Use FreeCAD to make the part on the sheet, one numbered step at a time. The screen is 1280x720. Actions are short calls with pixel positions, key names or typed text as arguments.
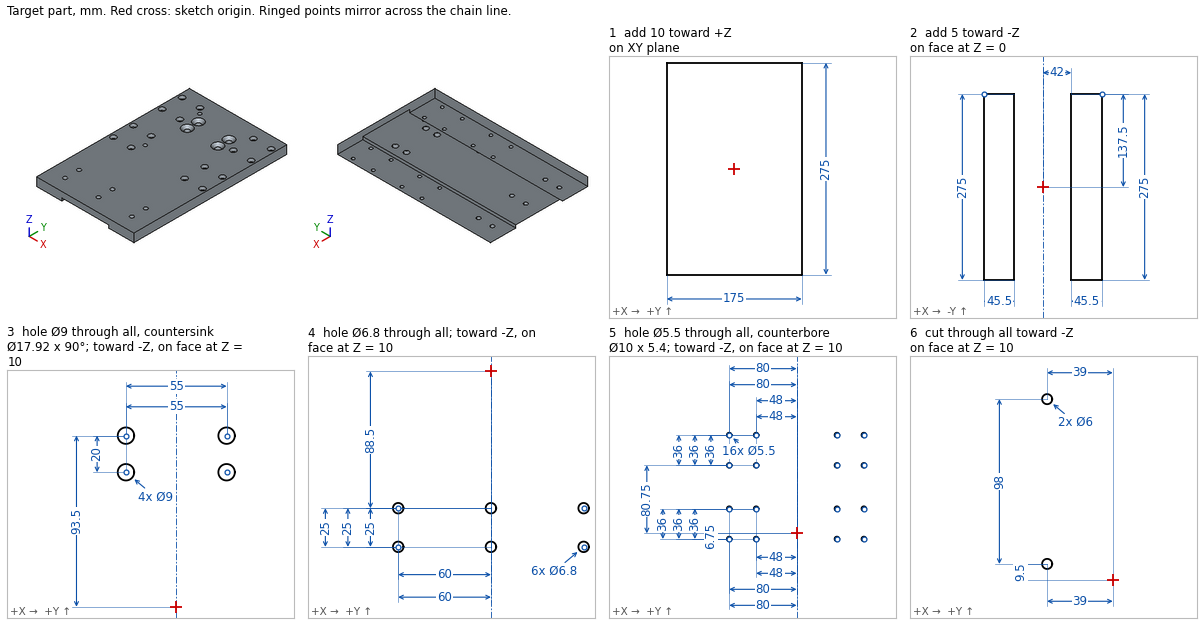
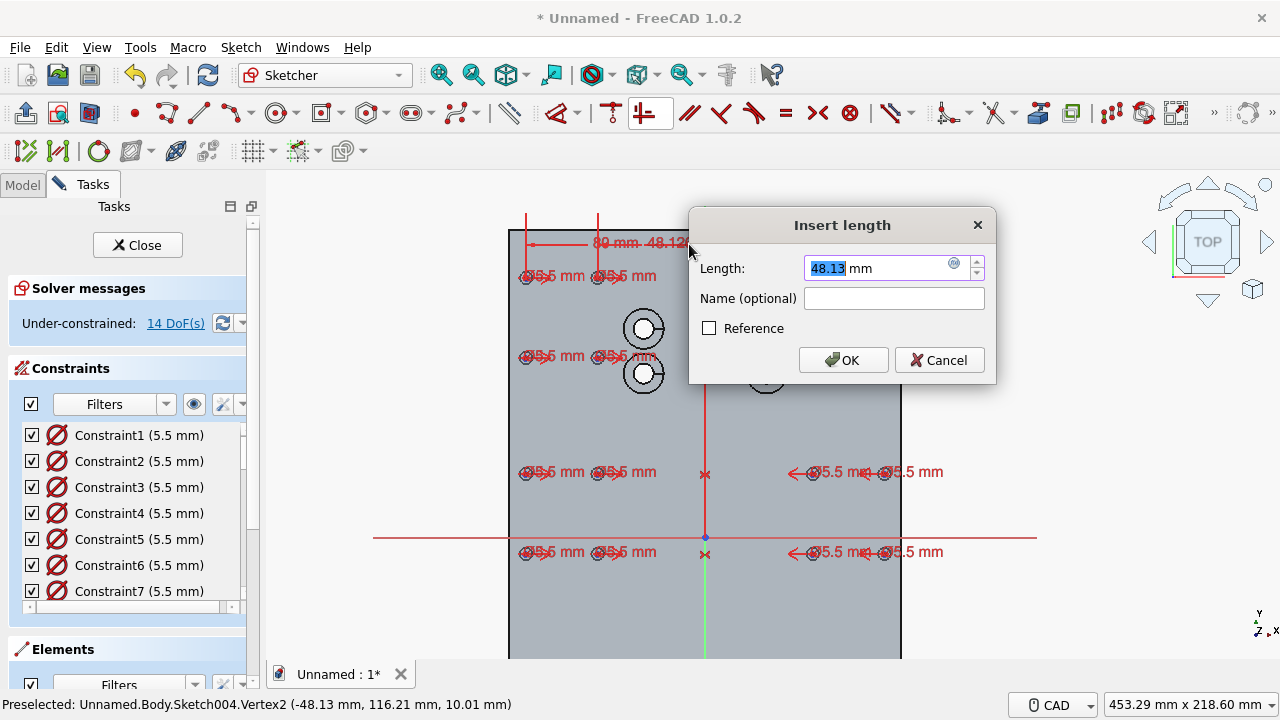
text(48)
key(Return)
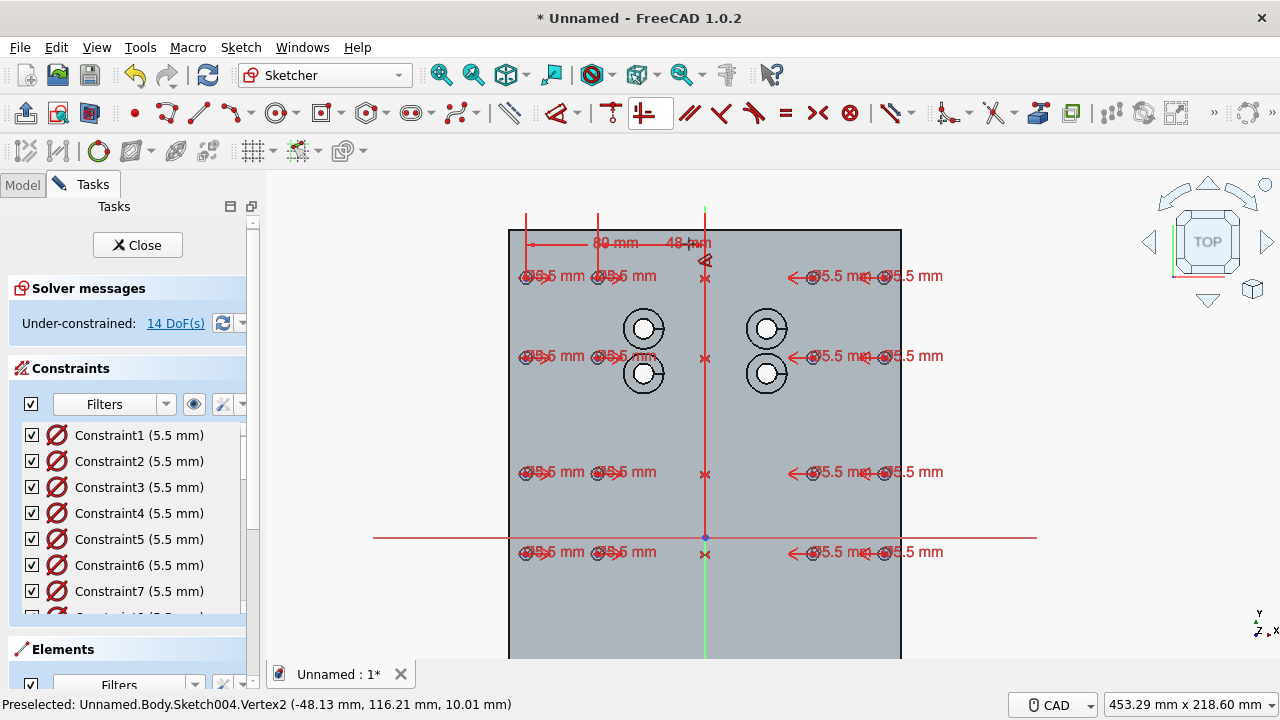
click(526, 358)
click(616, 572)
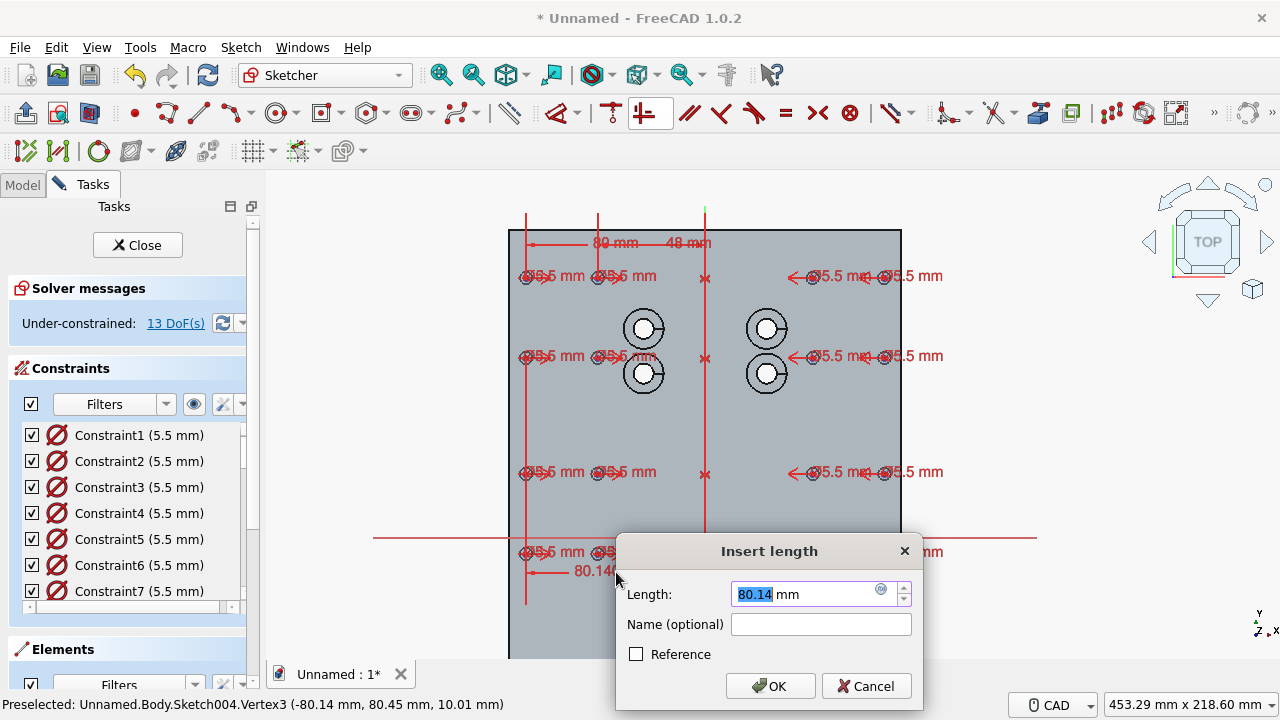
text(80)
key(Return)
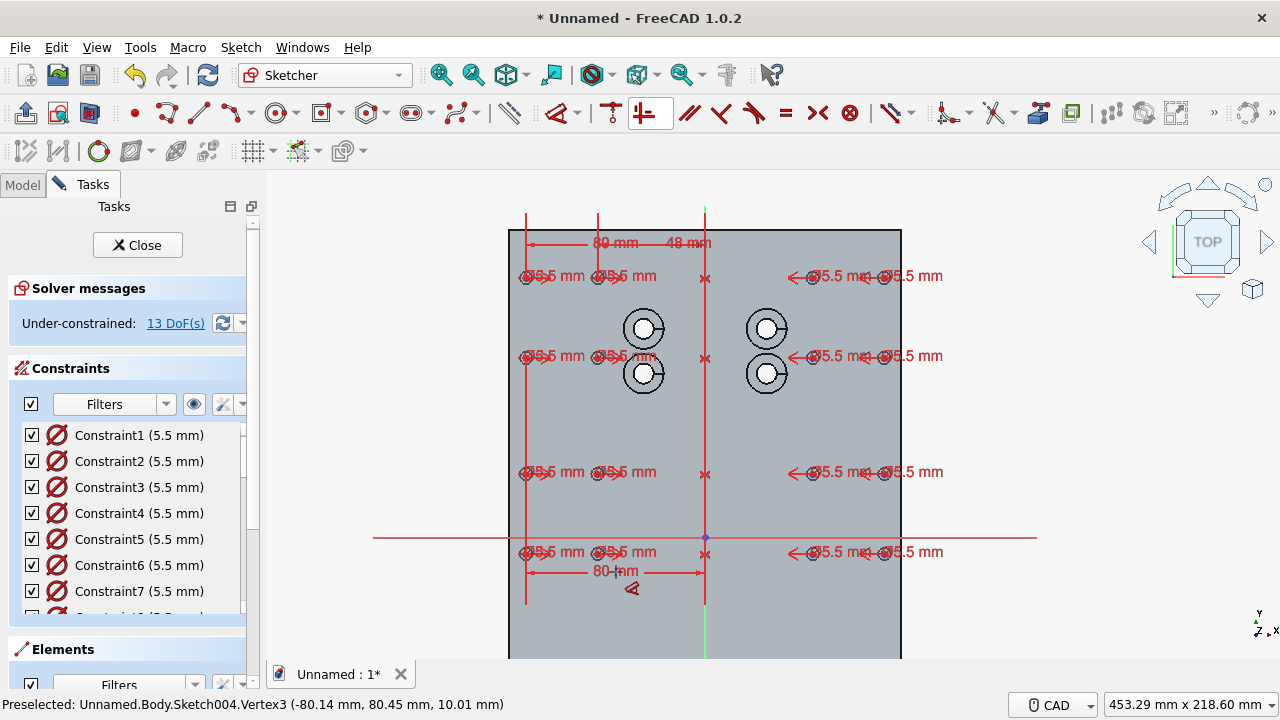
click(598, 358)
click(689, 572)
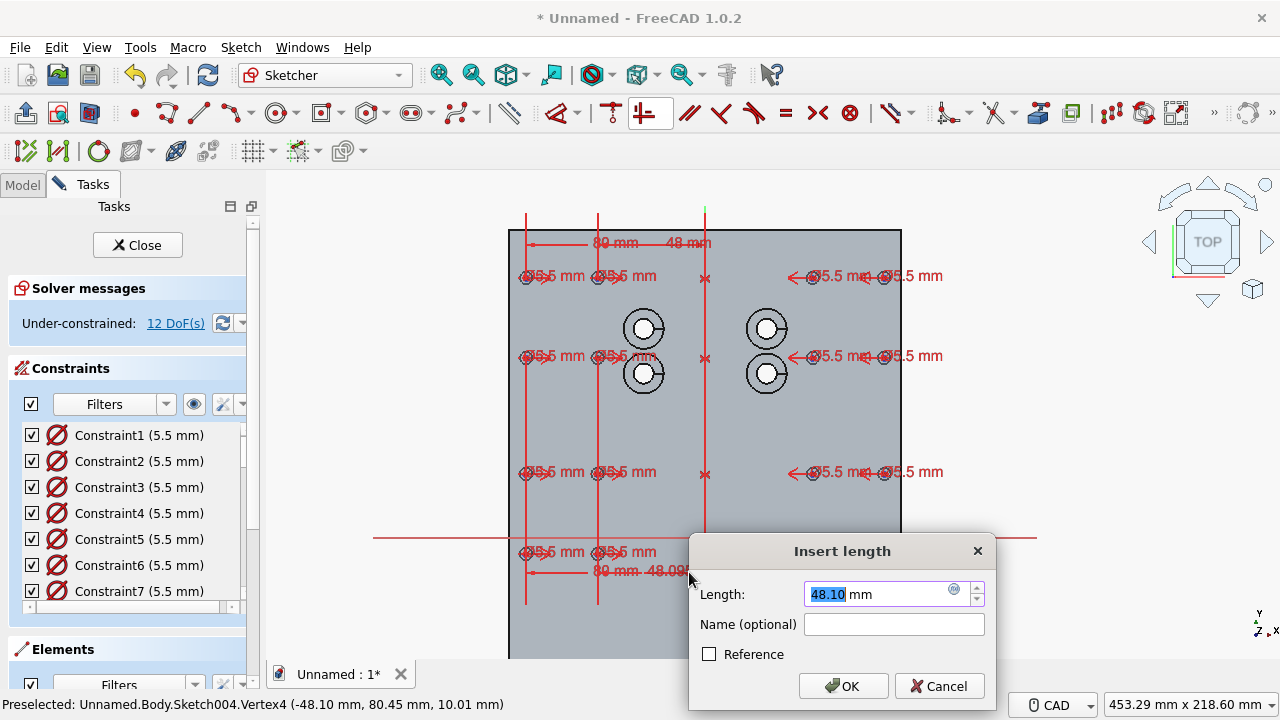
text(48)
key(Return)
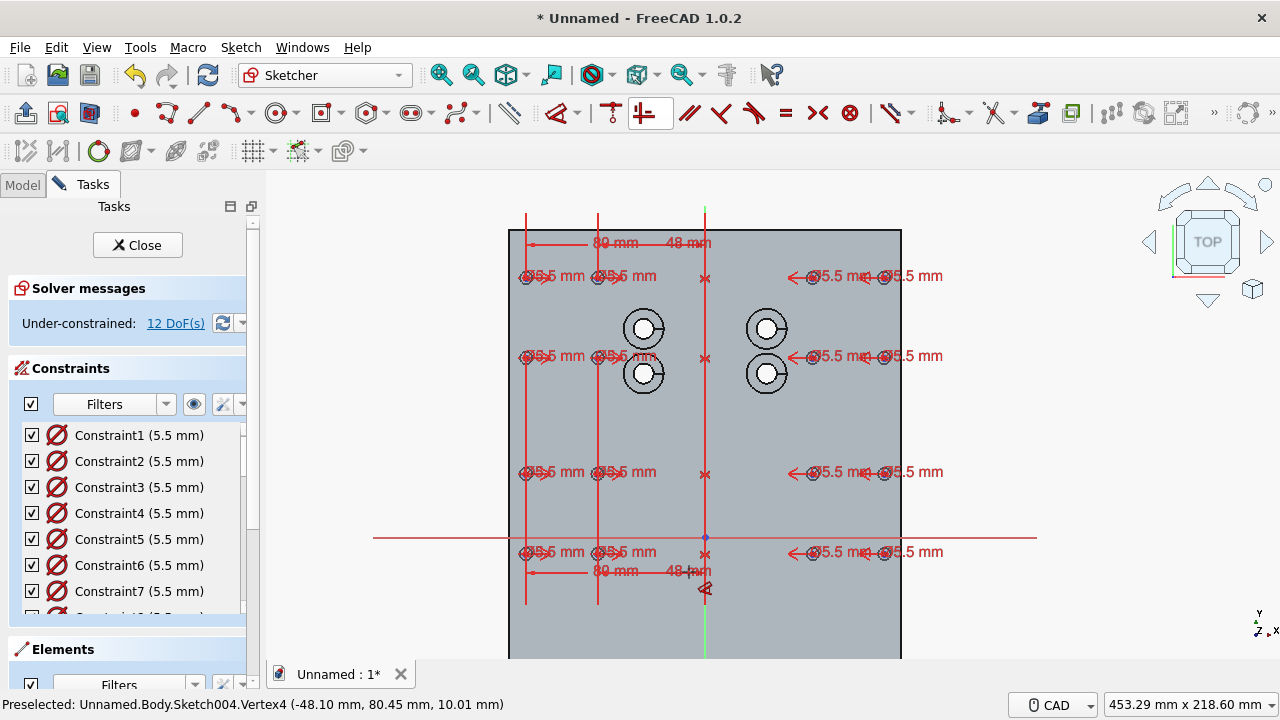
click(526, 474)
click(616, 440)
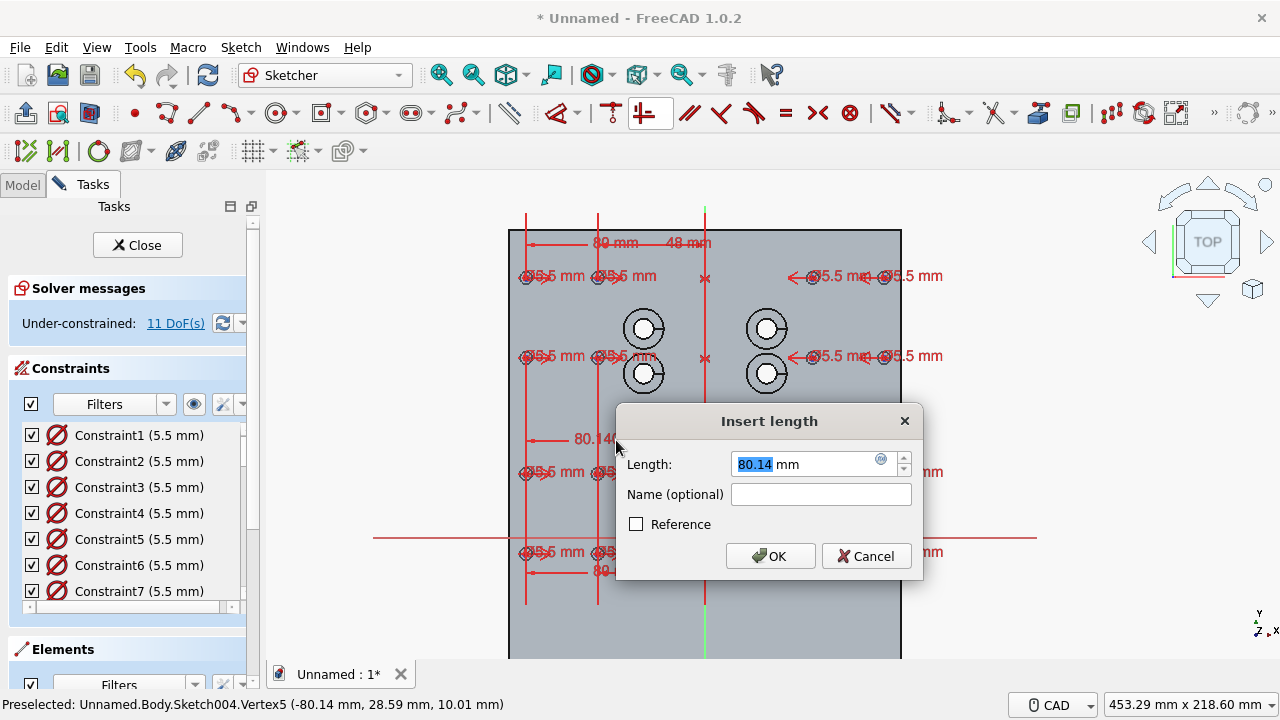
text(80)
key(Return)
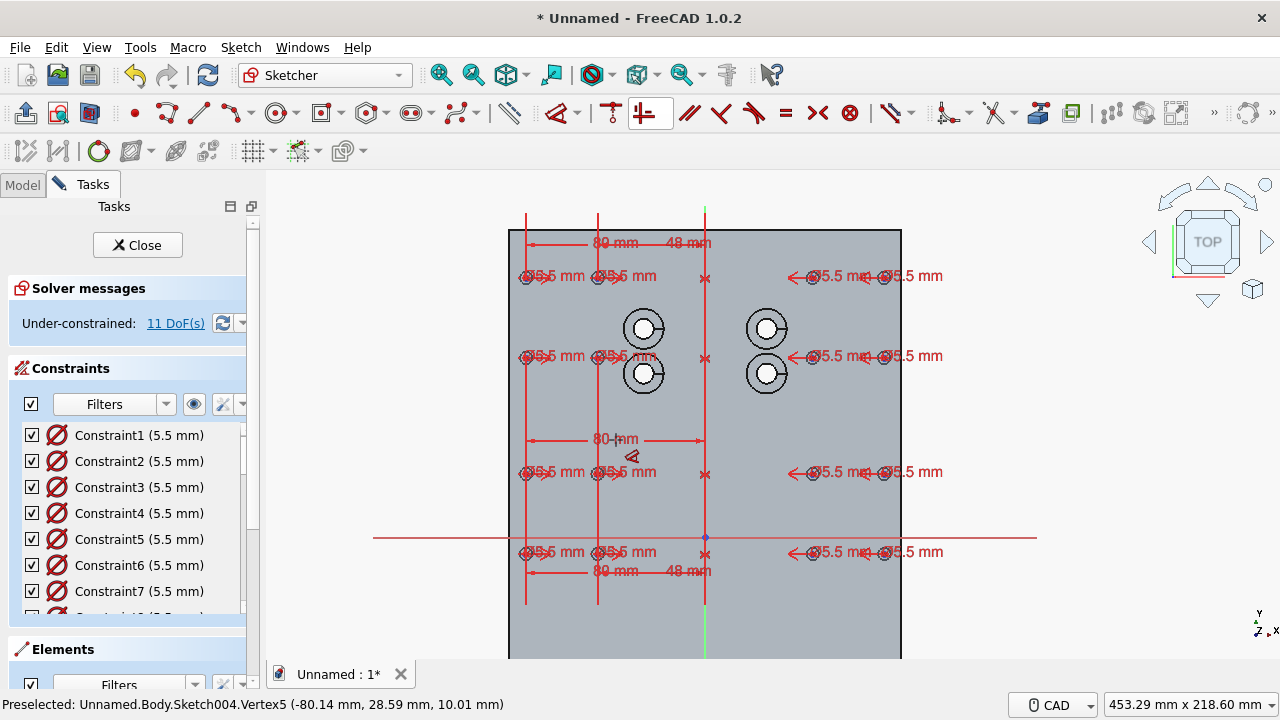
click(598, 474)
click(689, 440)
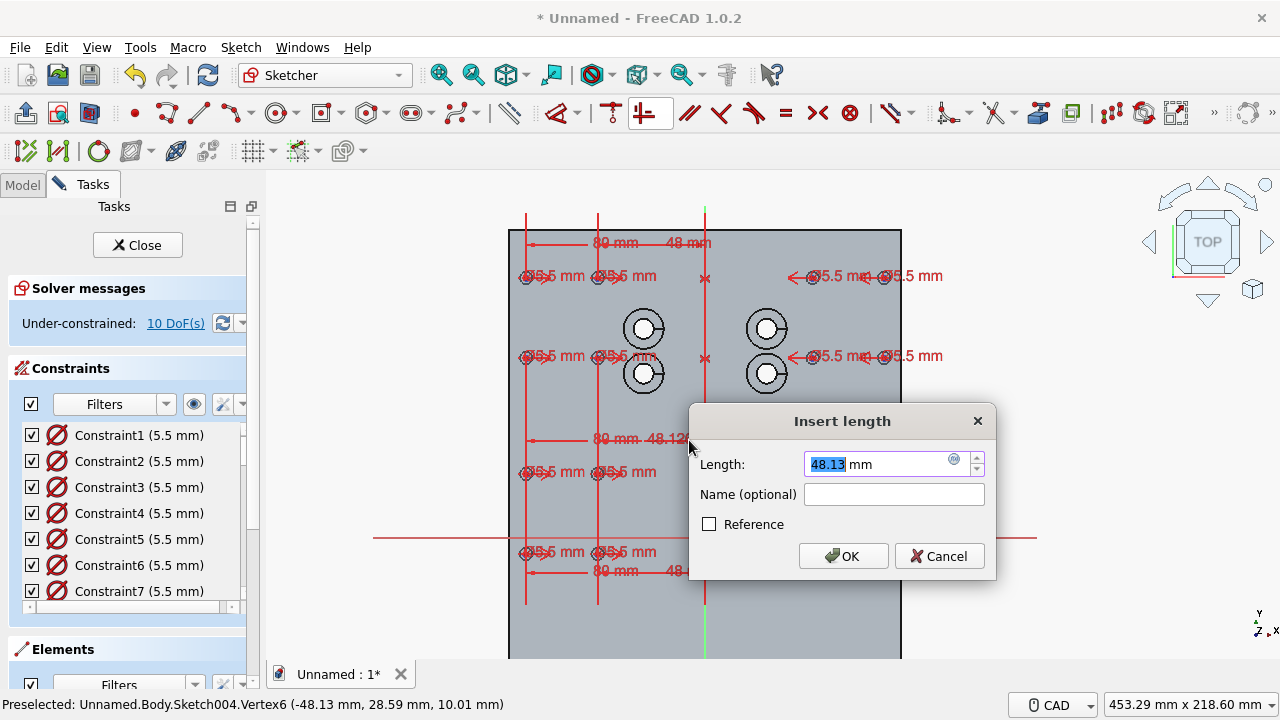
text(48)
key(Return)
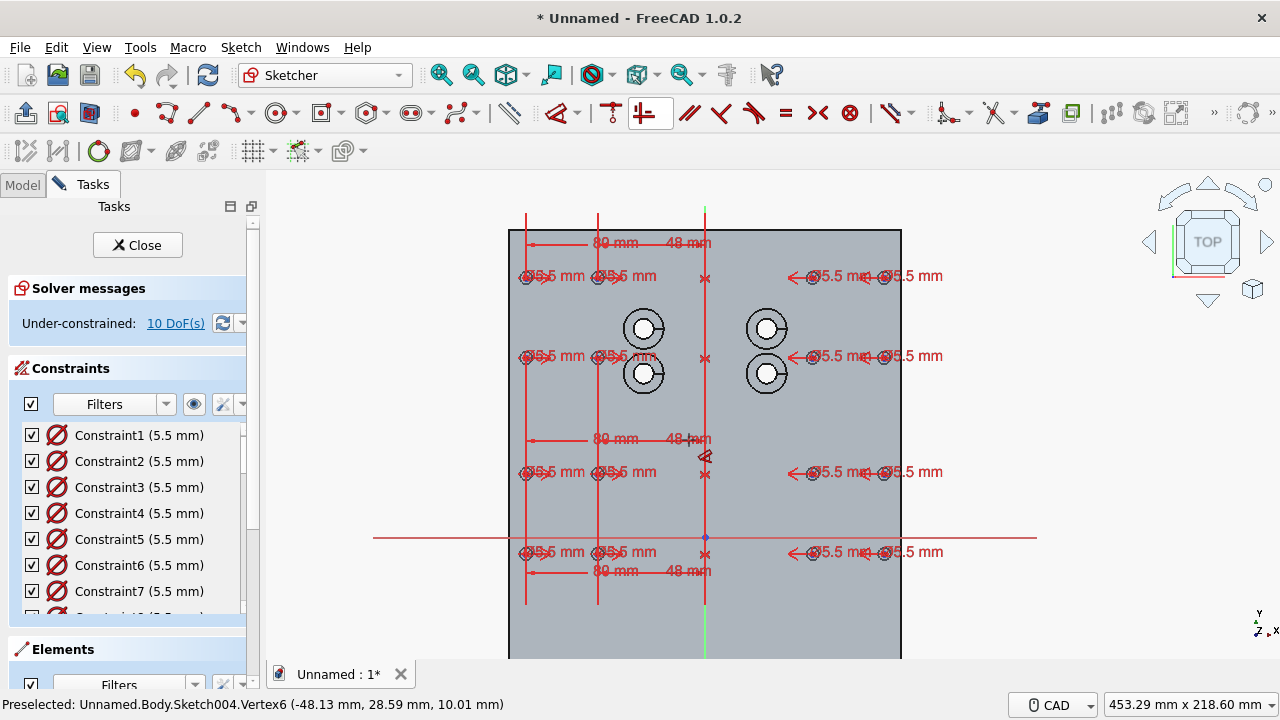
click(526, 554)
click(616, 504)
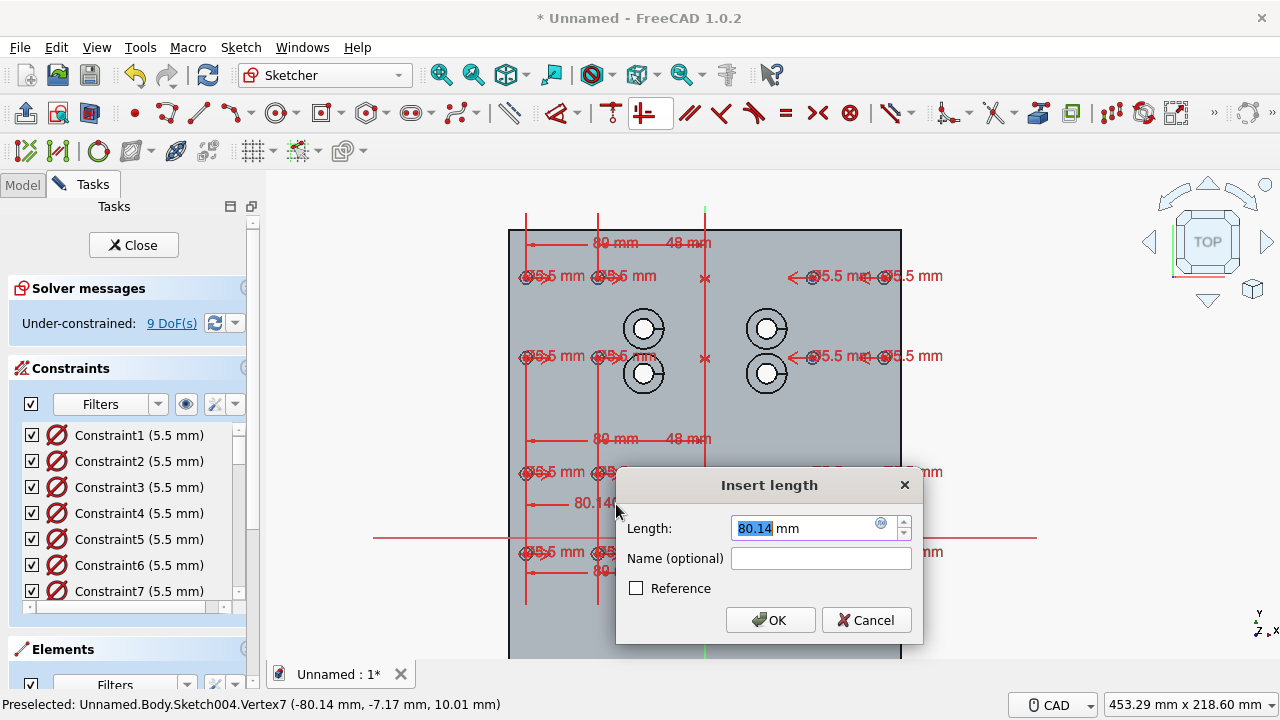
text(80)
key(Return)